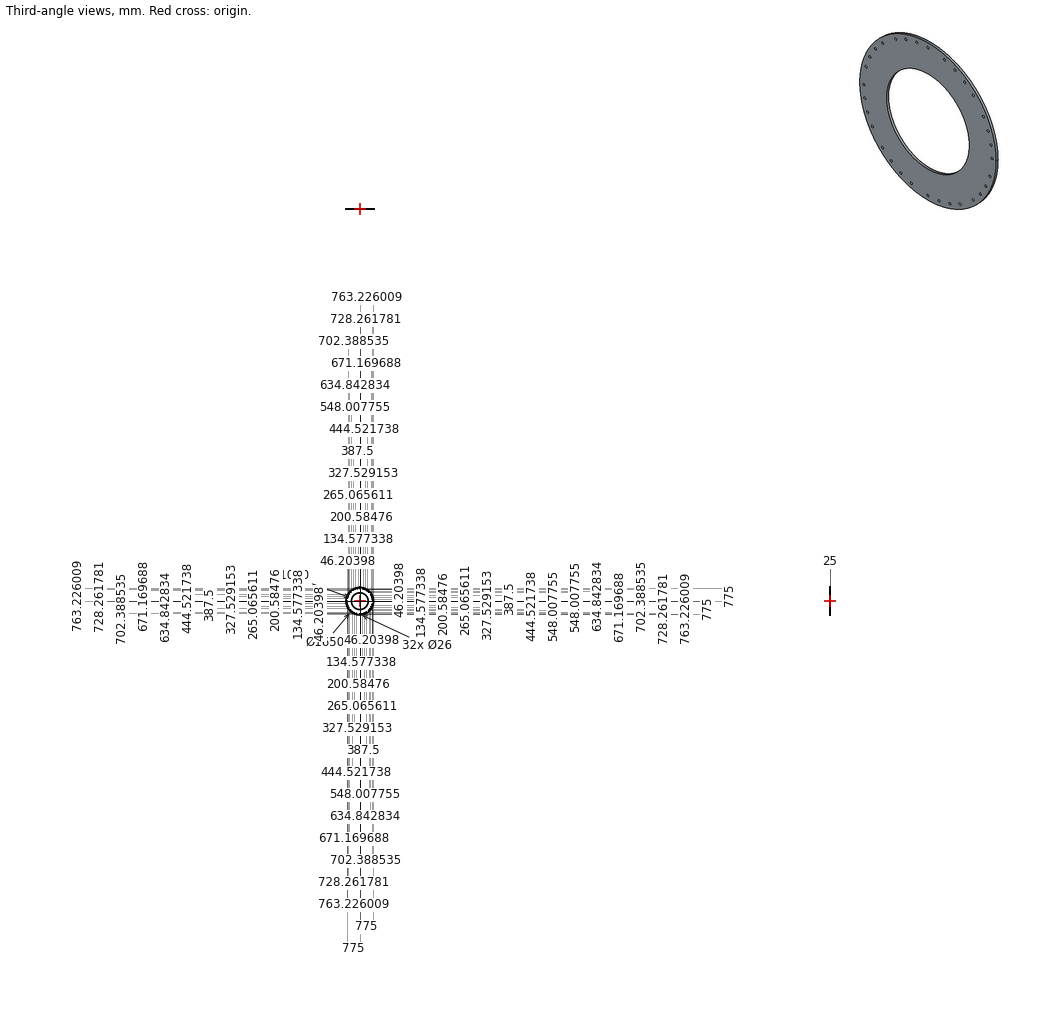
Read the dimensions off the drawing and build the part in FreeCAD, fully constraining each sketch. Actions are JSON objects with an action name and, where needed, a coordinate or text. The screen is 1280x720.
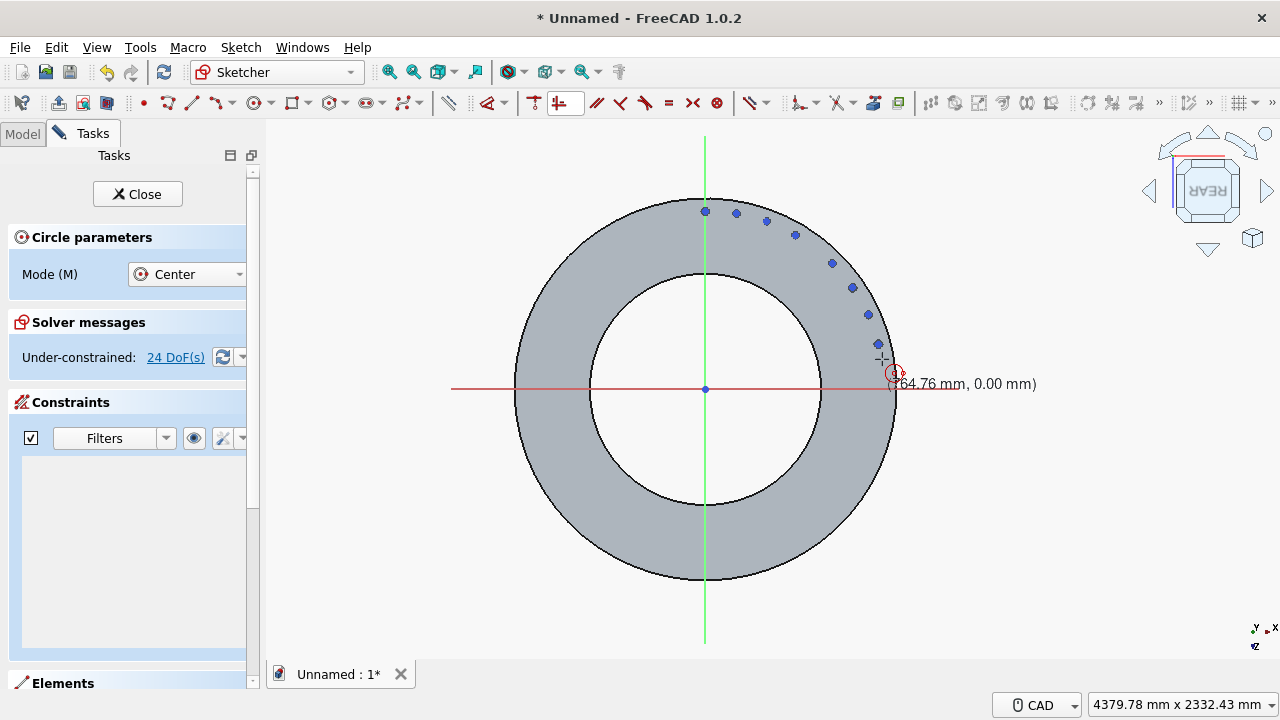
{"action": "left_click", "coordinate": [885, 389]}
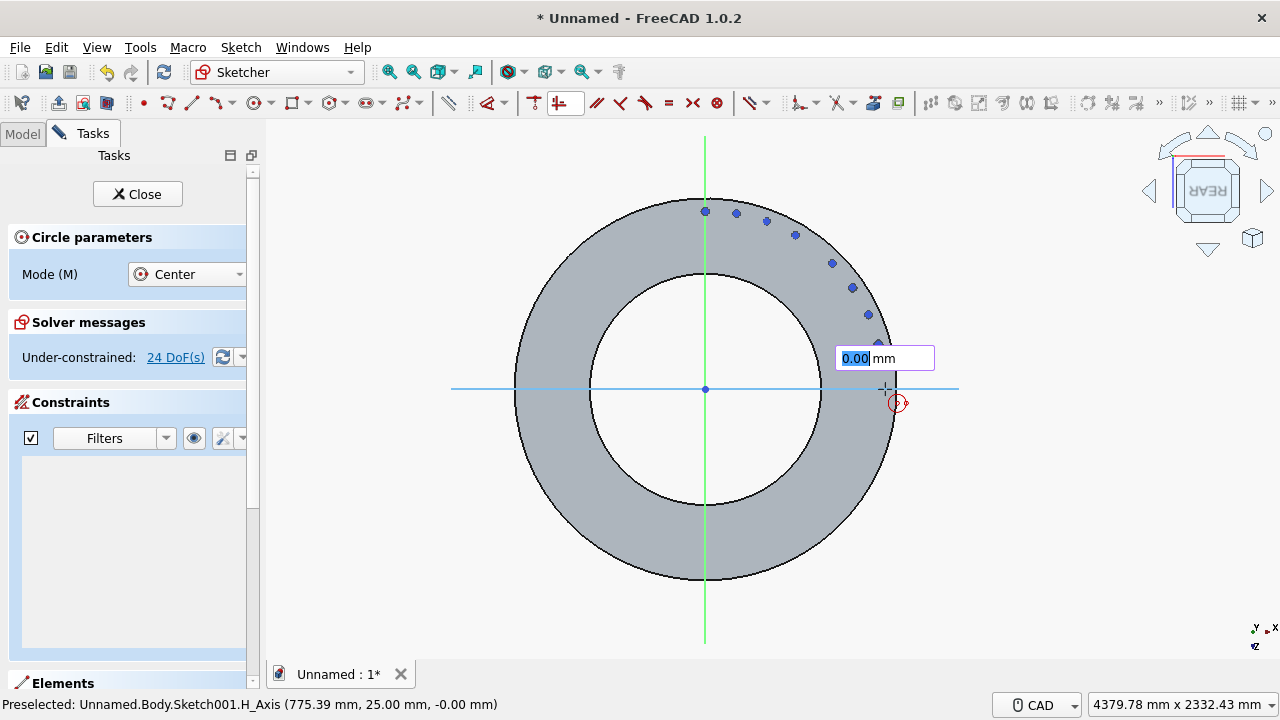
{"action": "scroll", "coordinate": [884, 392], "scroll_direction": "up", "scroll_amount": 9}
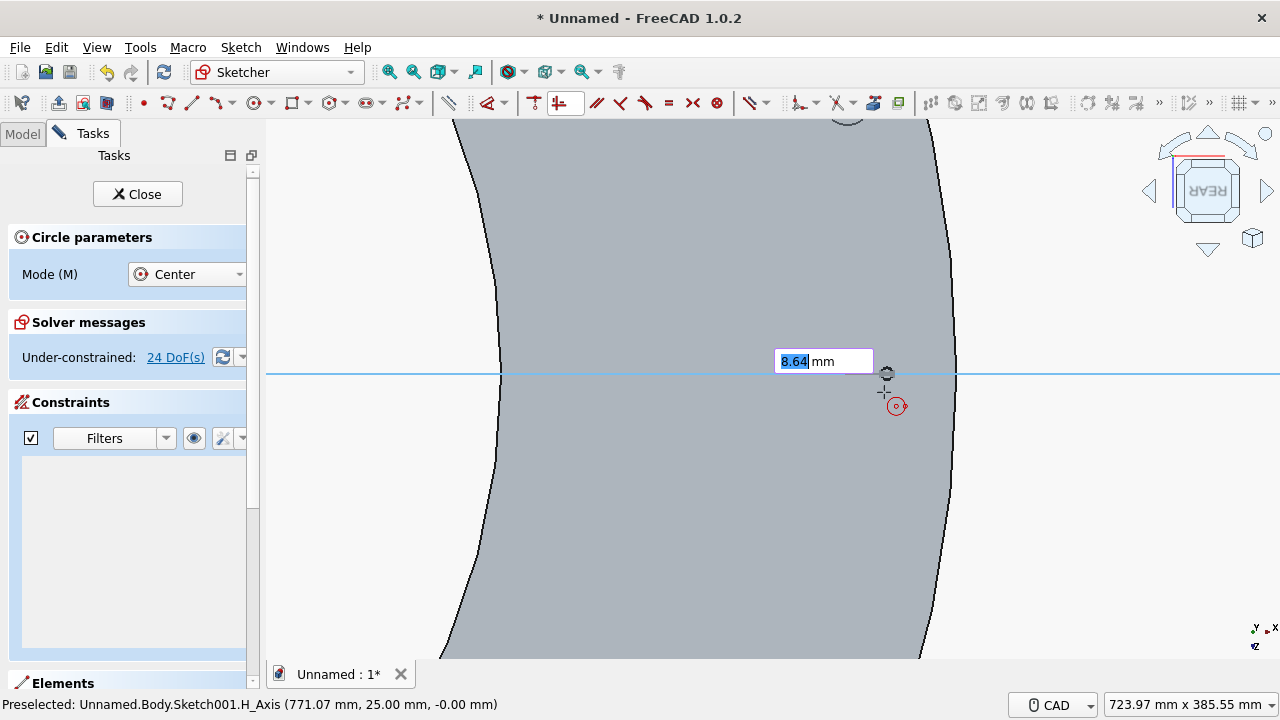
{"action": "left_click", "coordinate": [880, 391]}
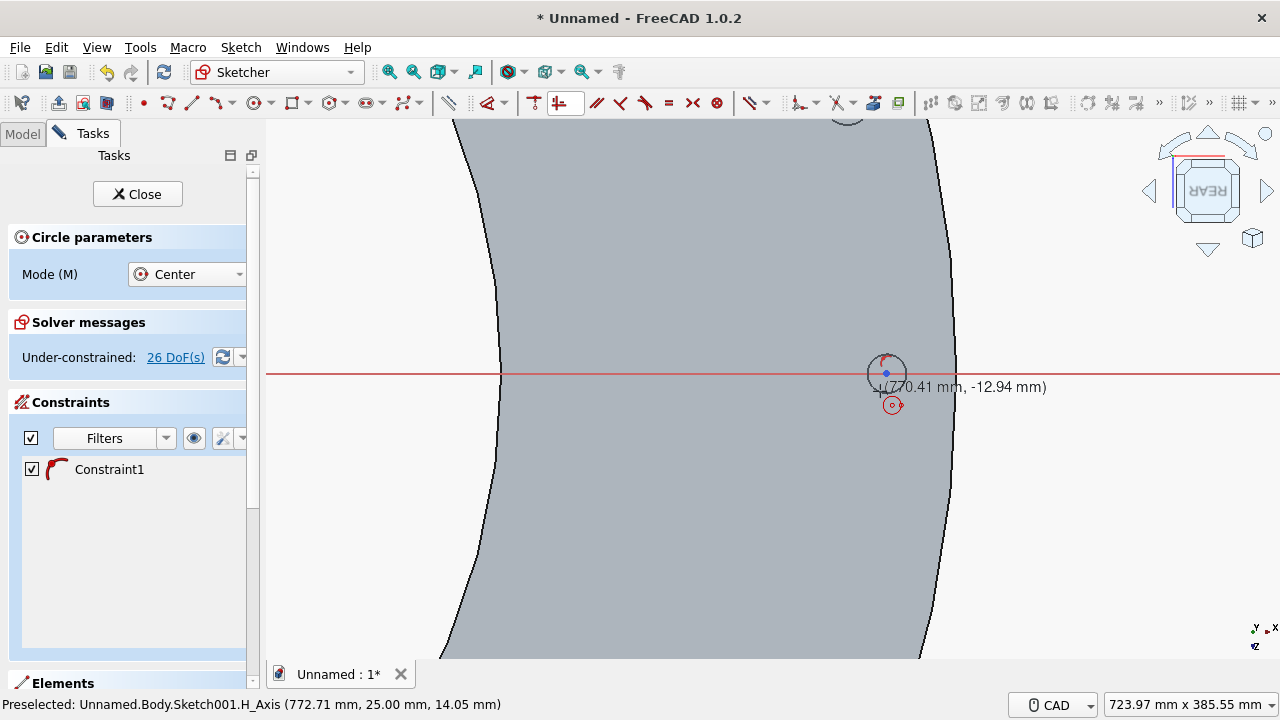
{"action": "scroll", "coordinate": [870, 562], "scroll_direction": "up", "scroll_amount": 2}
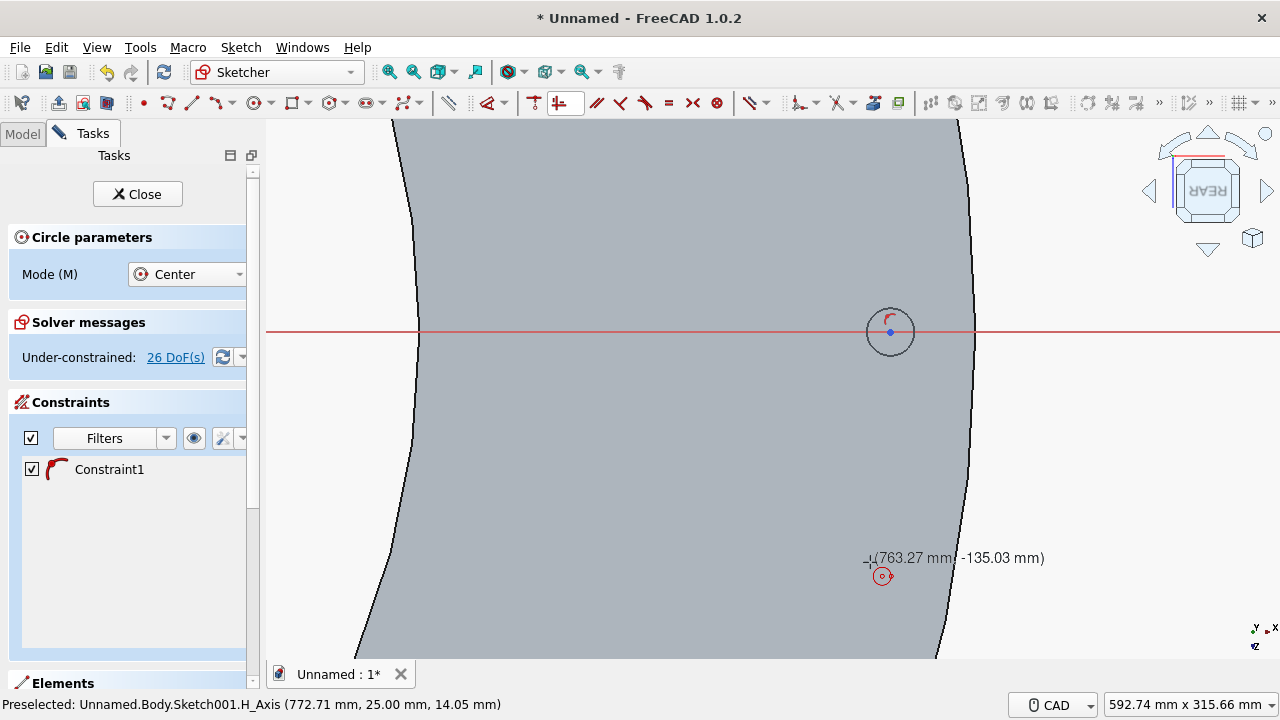
{"action": "scroll", "coordinate": [883, 402], "scroll_direction": "down", "scroll_amount": 11}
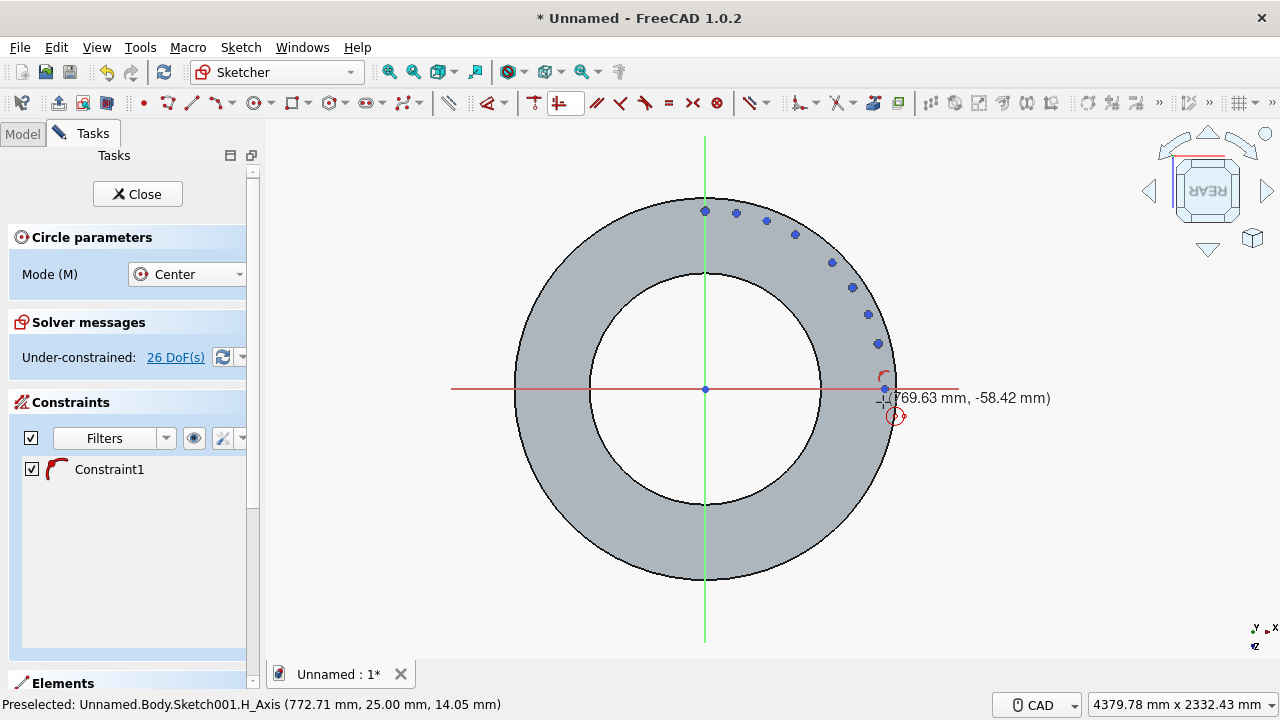
{"action": "left_click", "coordinate": [882, 420]}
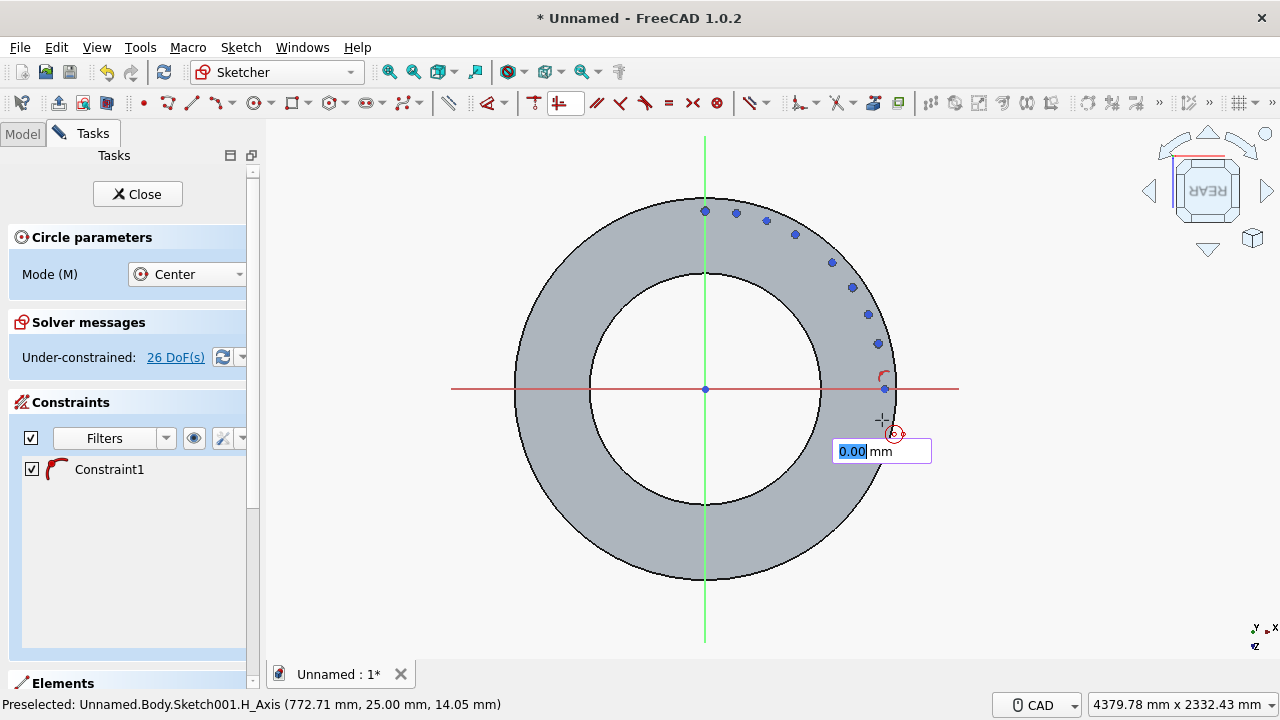
{"action": "scroll", "coordinate": [884, 418], "scroll_direction": "up", "scroll_amount": 9}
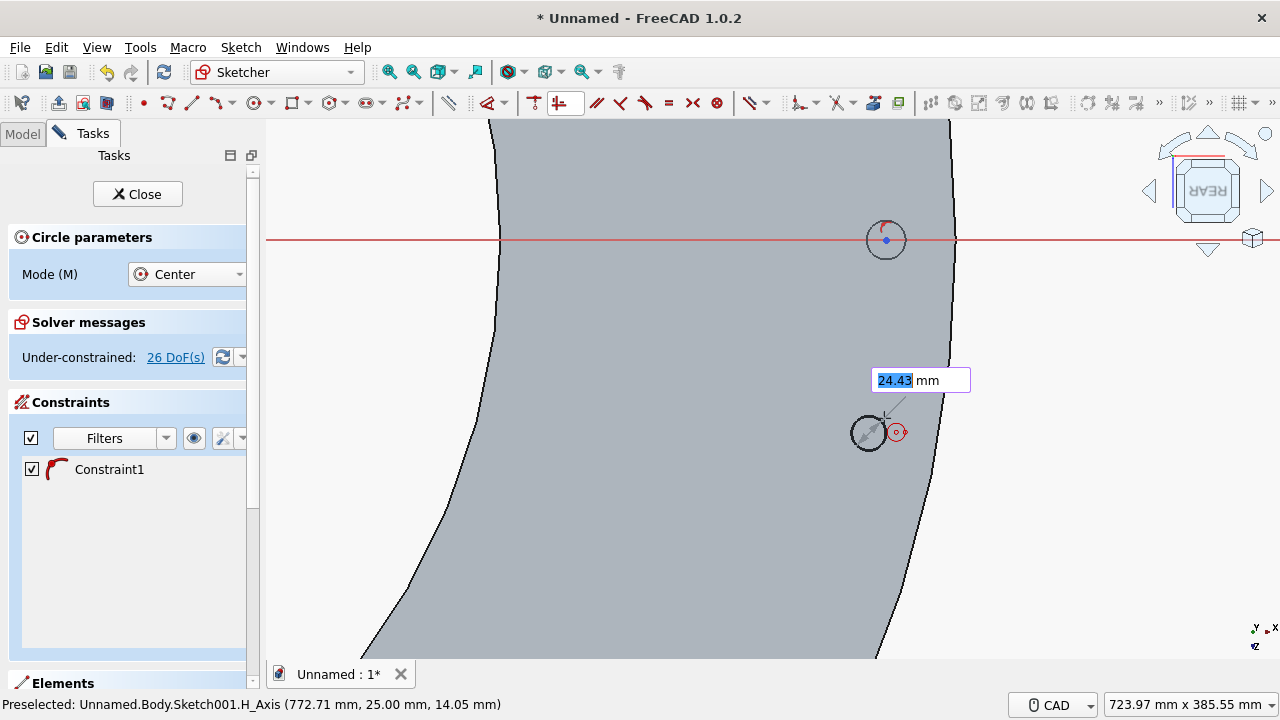
{"action": "left_click", "coordinate": [882, 416]}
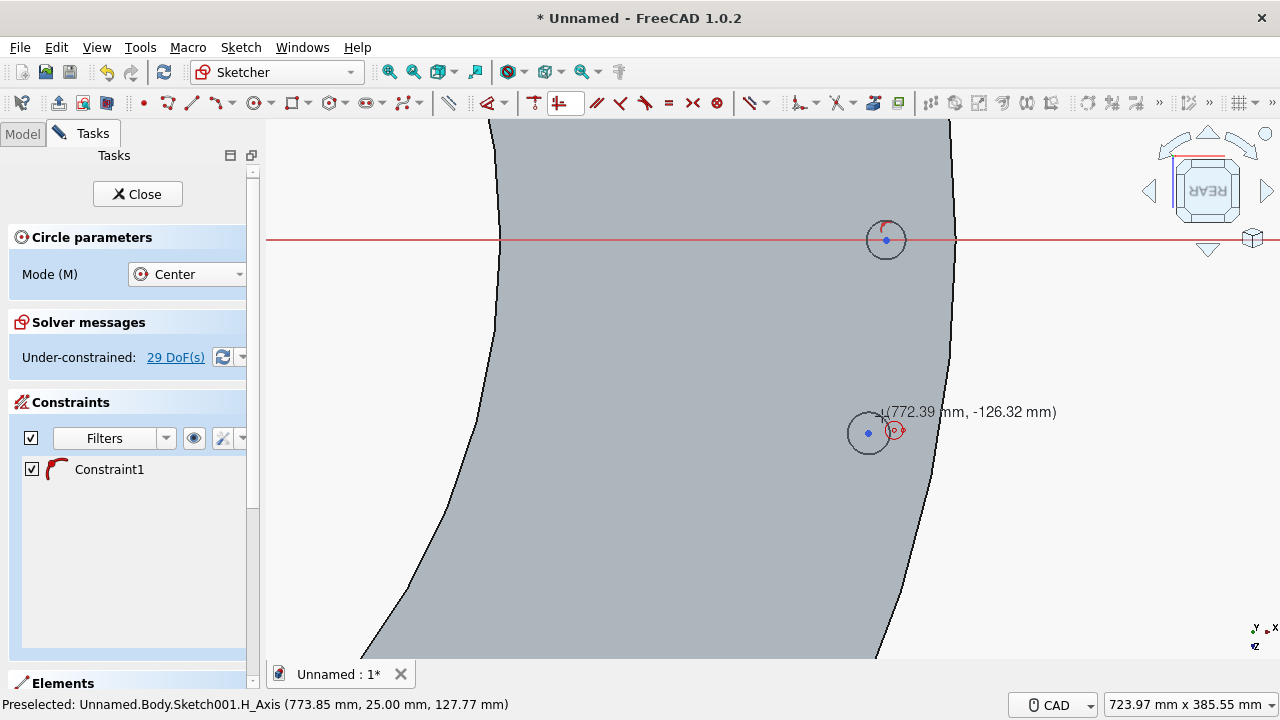
{"action": "scroll", "coordinate": [820, 611], "scroll_direction": "up", "scroll_amount": 2}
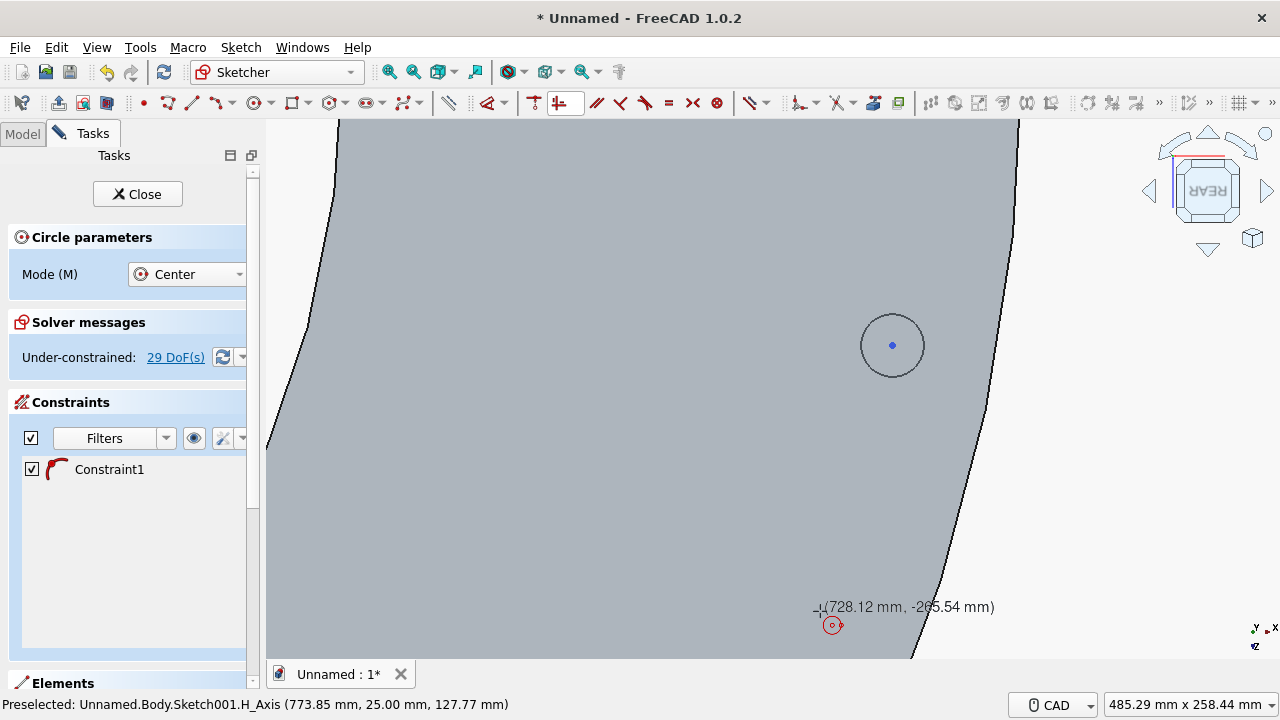
{"action": "scroll", "coordinate": [880, 430], "scroll_direction": "down", "scroll_amount": 11}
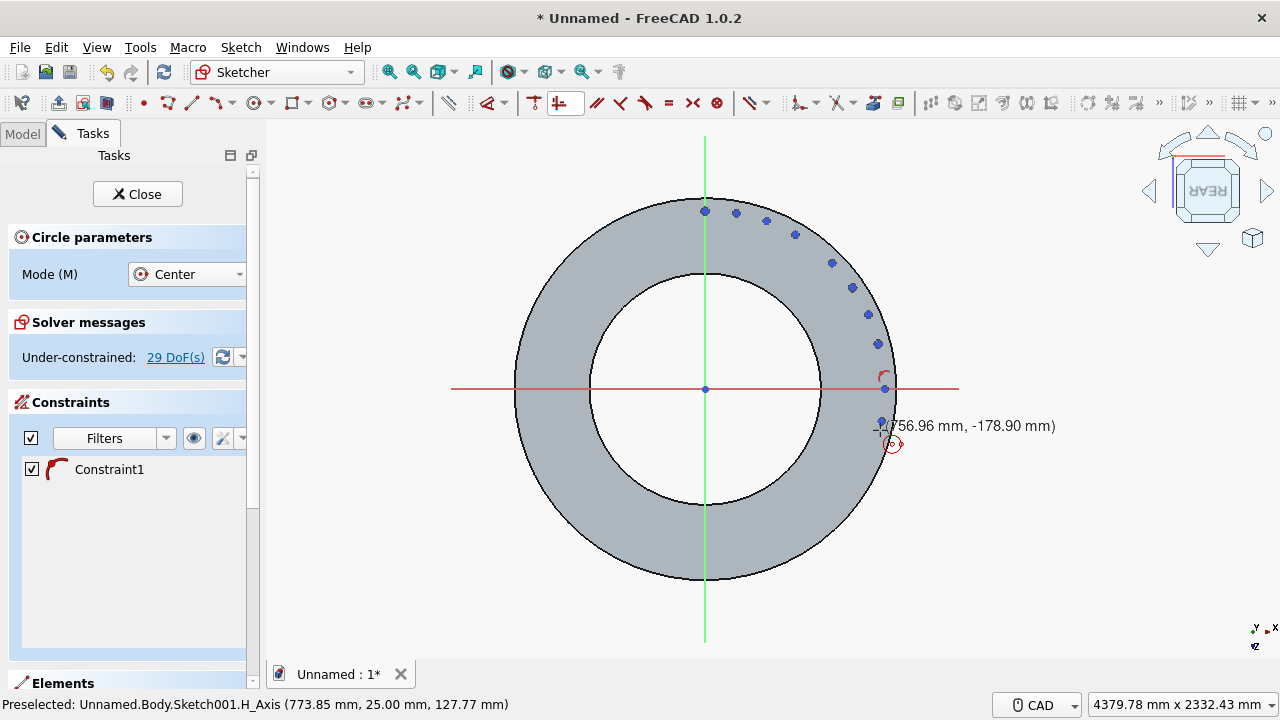
{"action": "left_click", "coordinate": [874, 451]}